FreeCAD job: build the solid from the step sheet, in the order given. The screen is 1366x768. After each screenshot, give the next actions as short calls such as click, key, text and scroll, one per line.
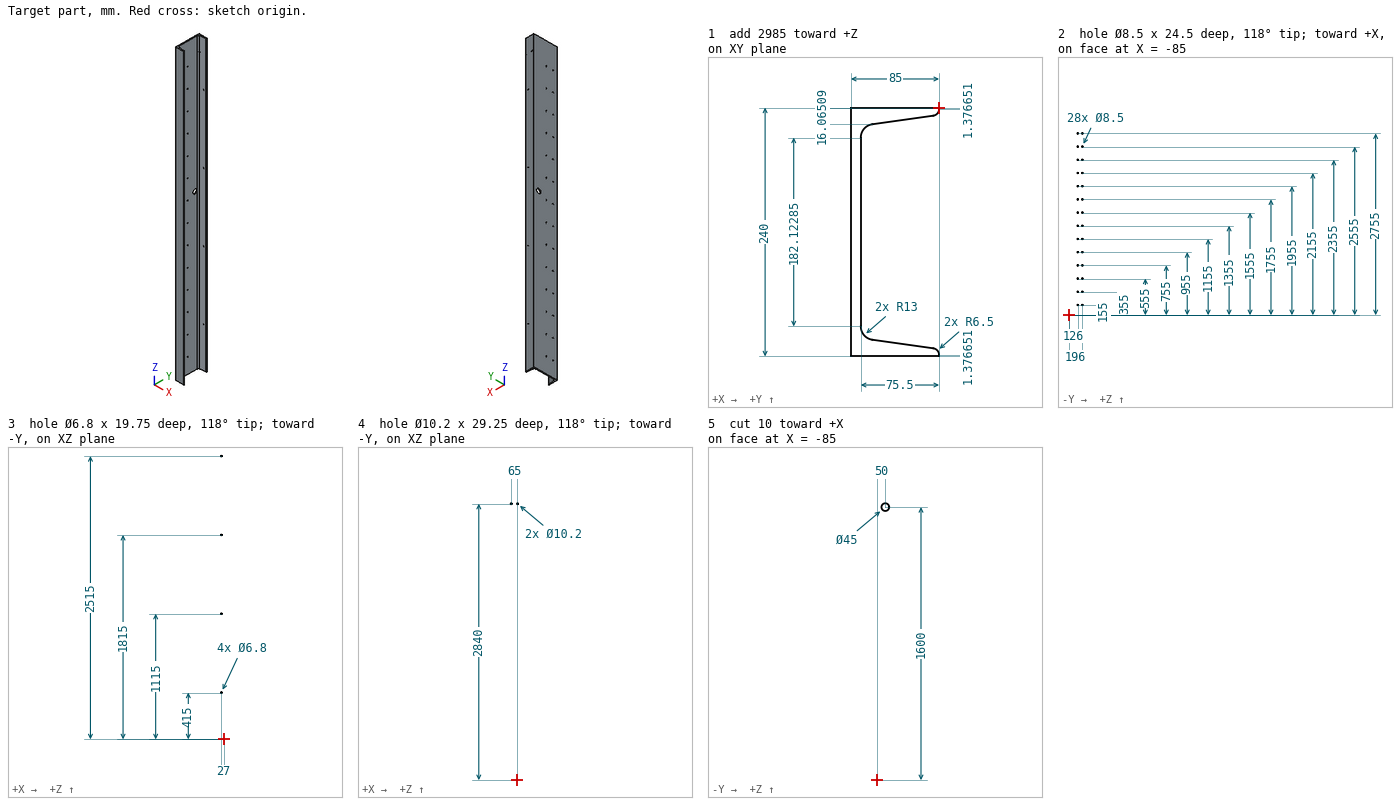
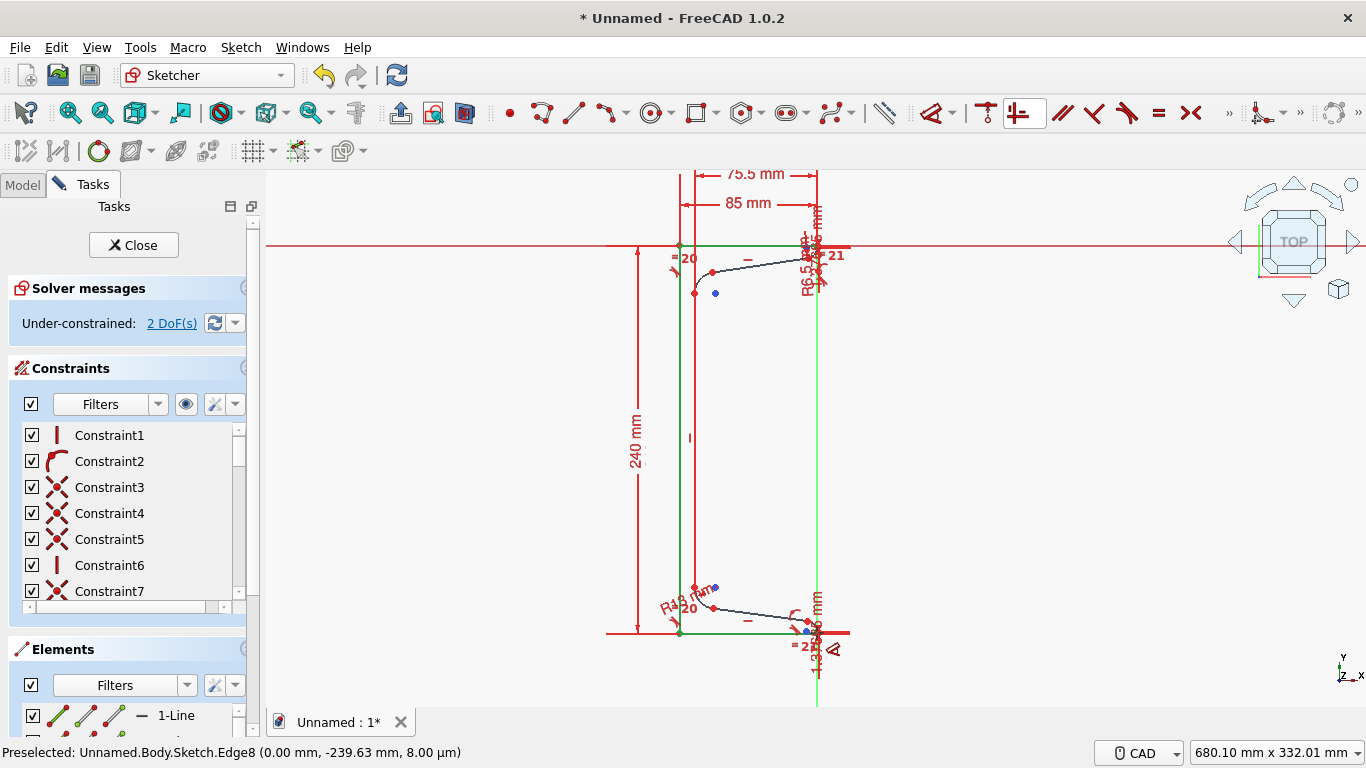
click(695, 499)
click(661, 373)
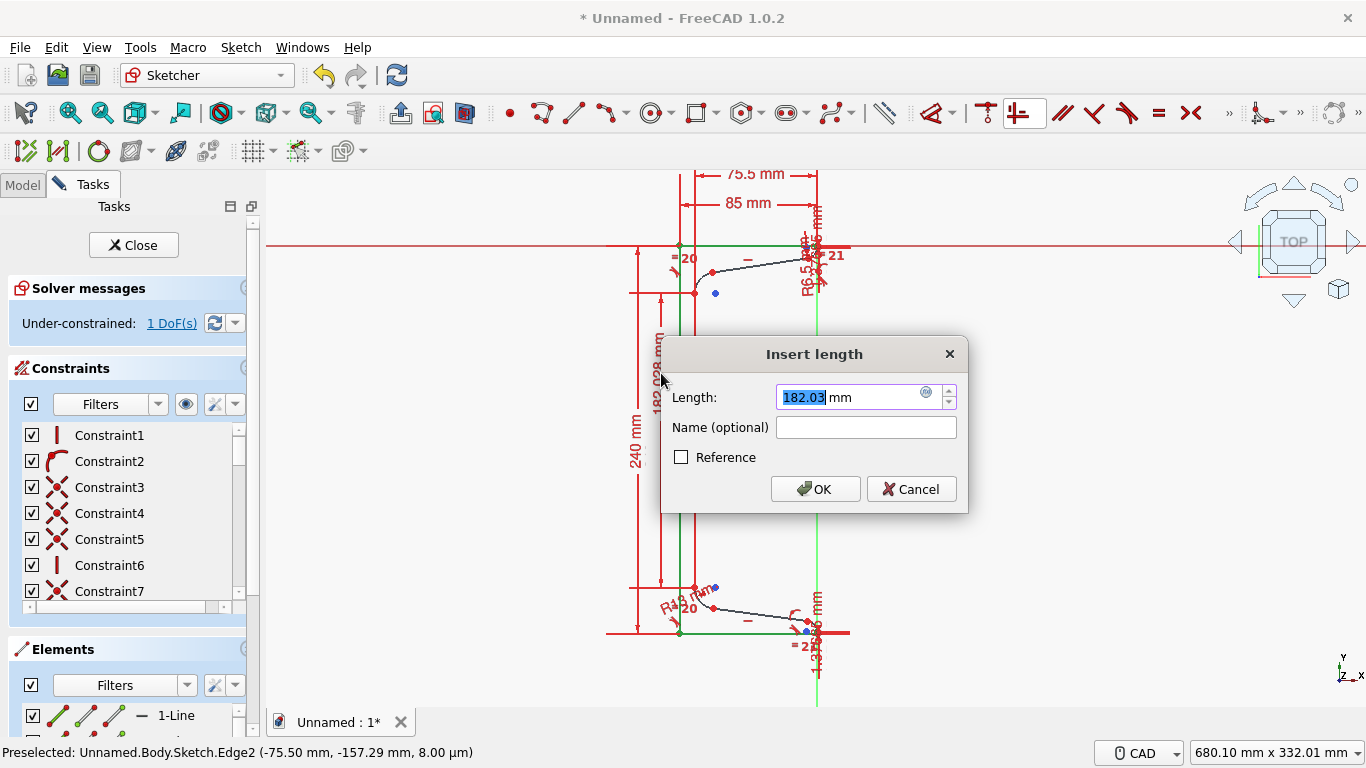
text(182.12285)
key(Return)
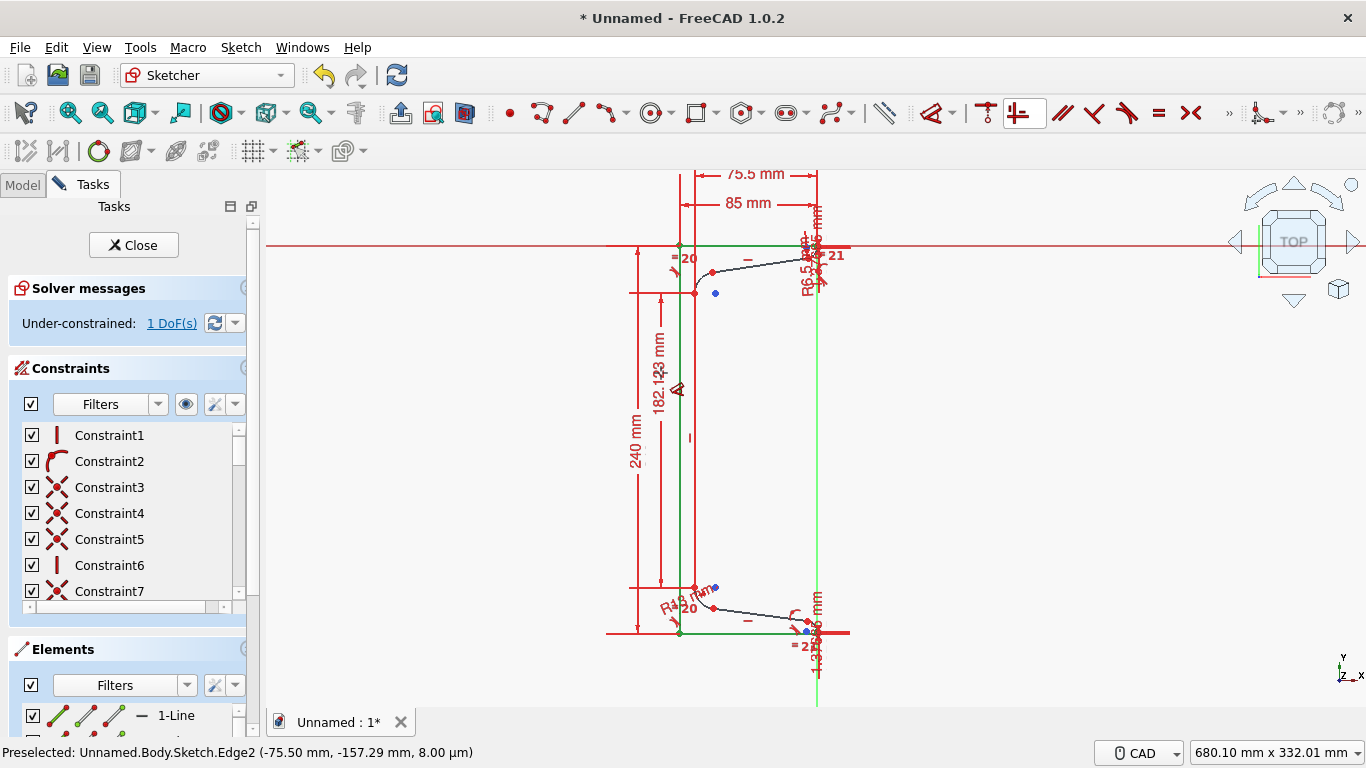
scroll(713, 273, up, 3)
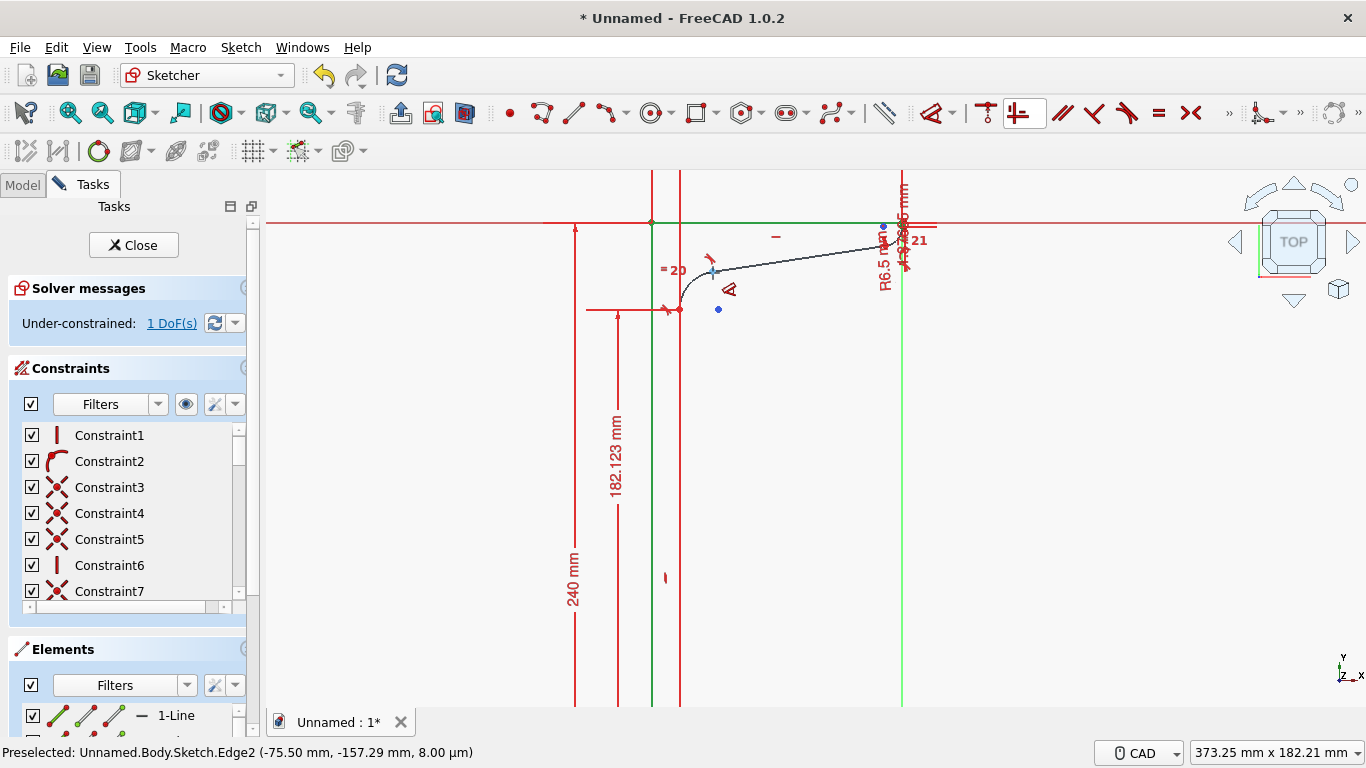
click(712, 272)
click(678, 247)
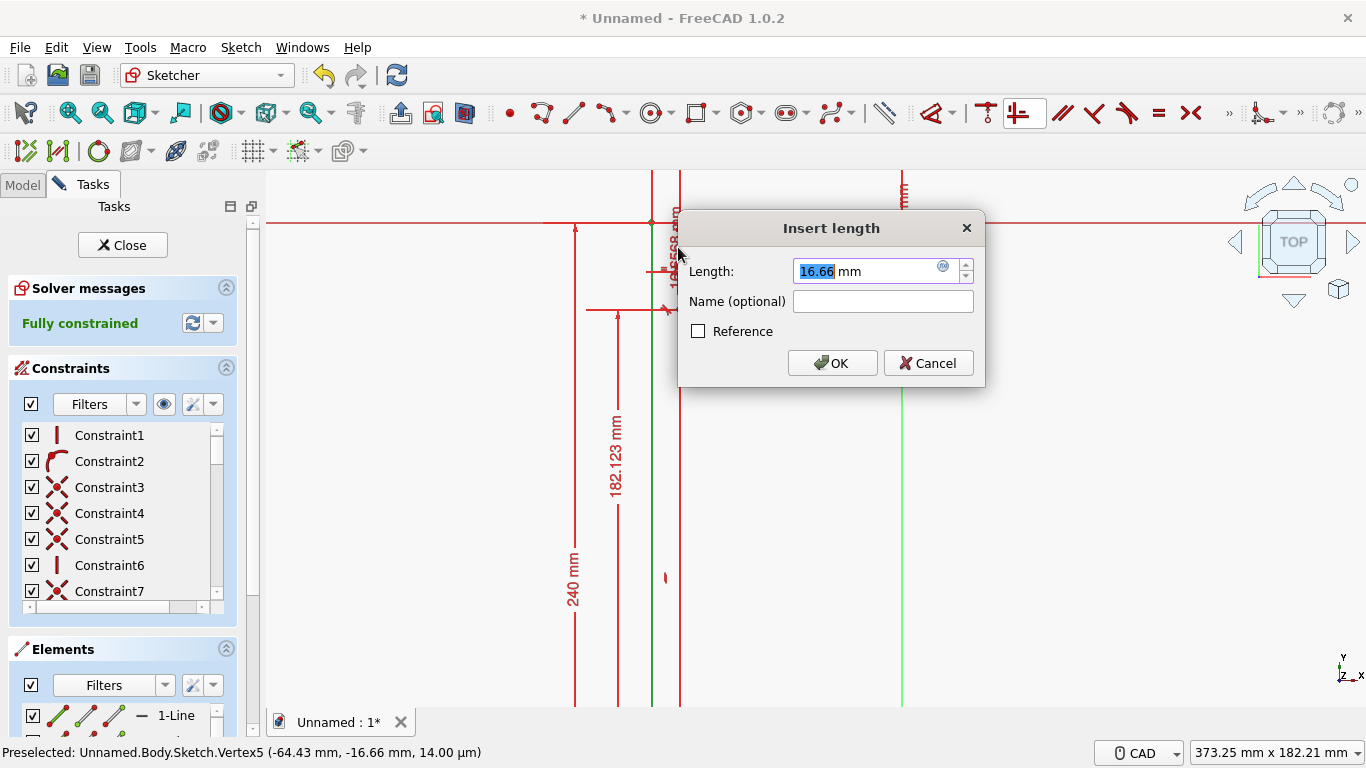
text(16.06509)
key(Return)
key(Escape)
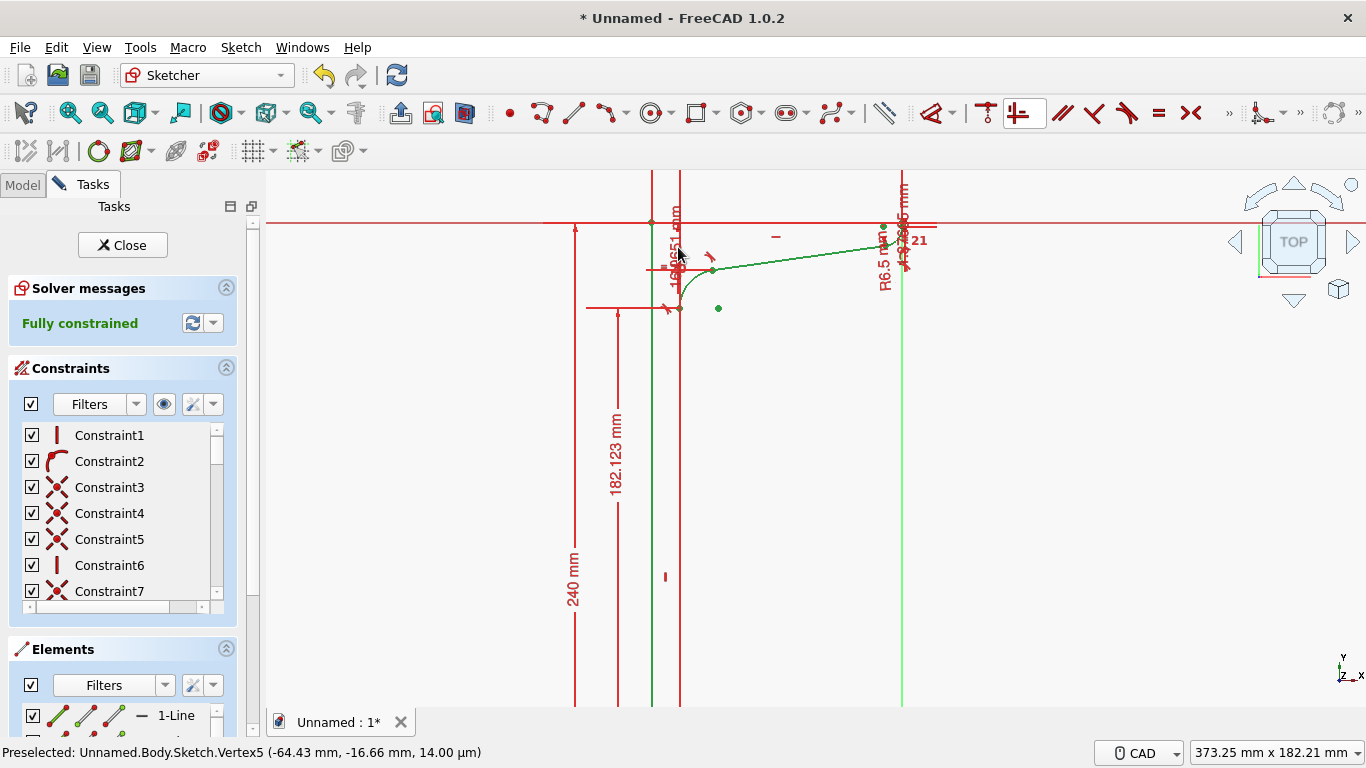
click(123, 245)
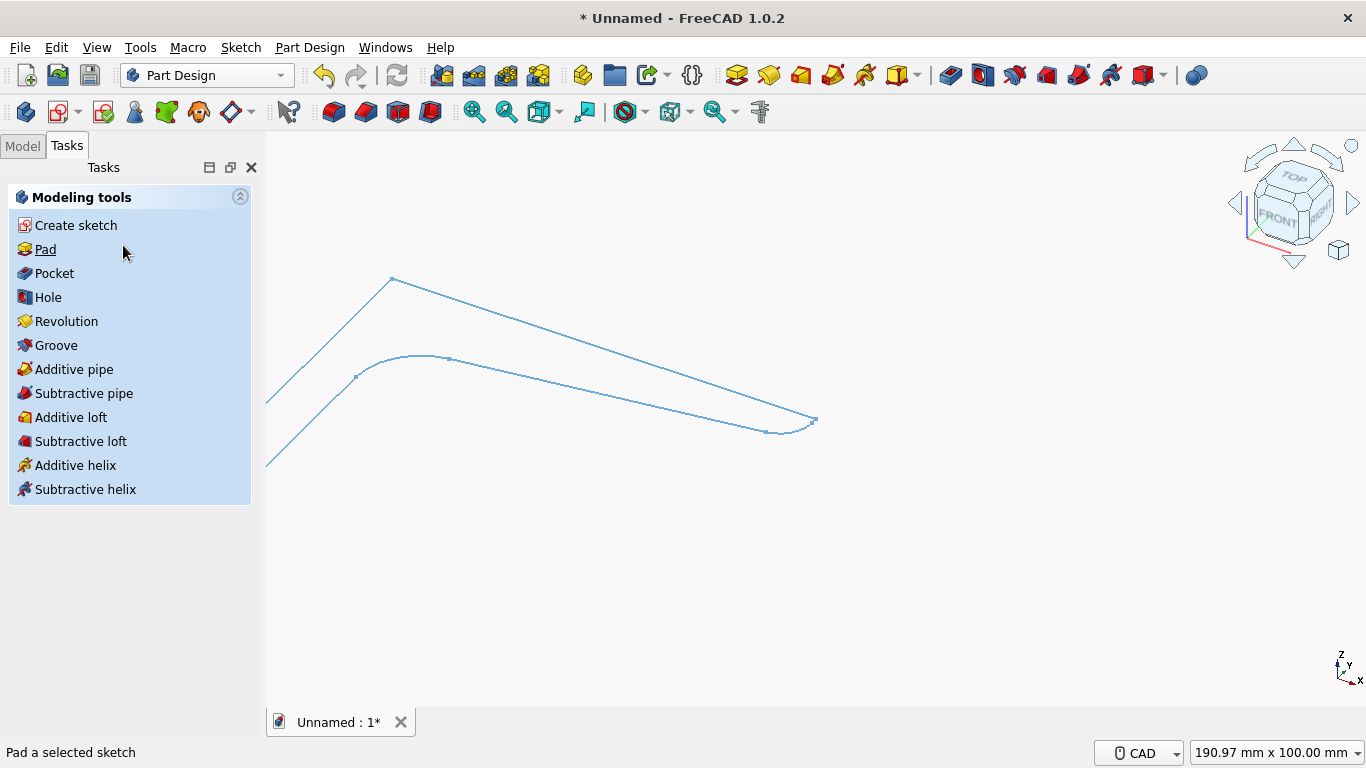
click(738, 76)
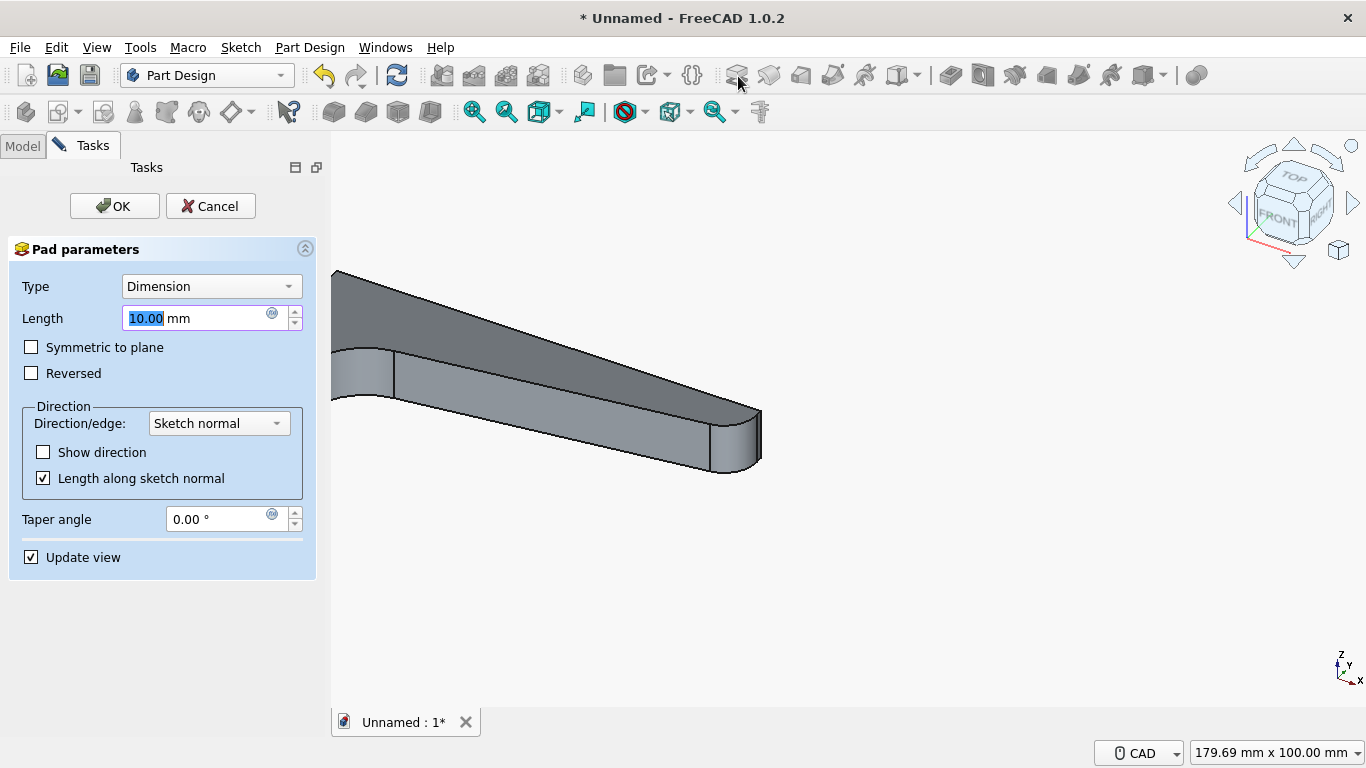
text(2985)
key(Tab)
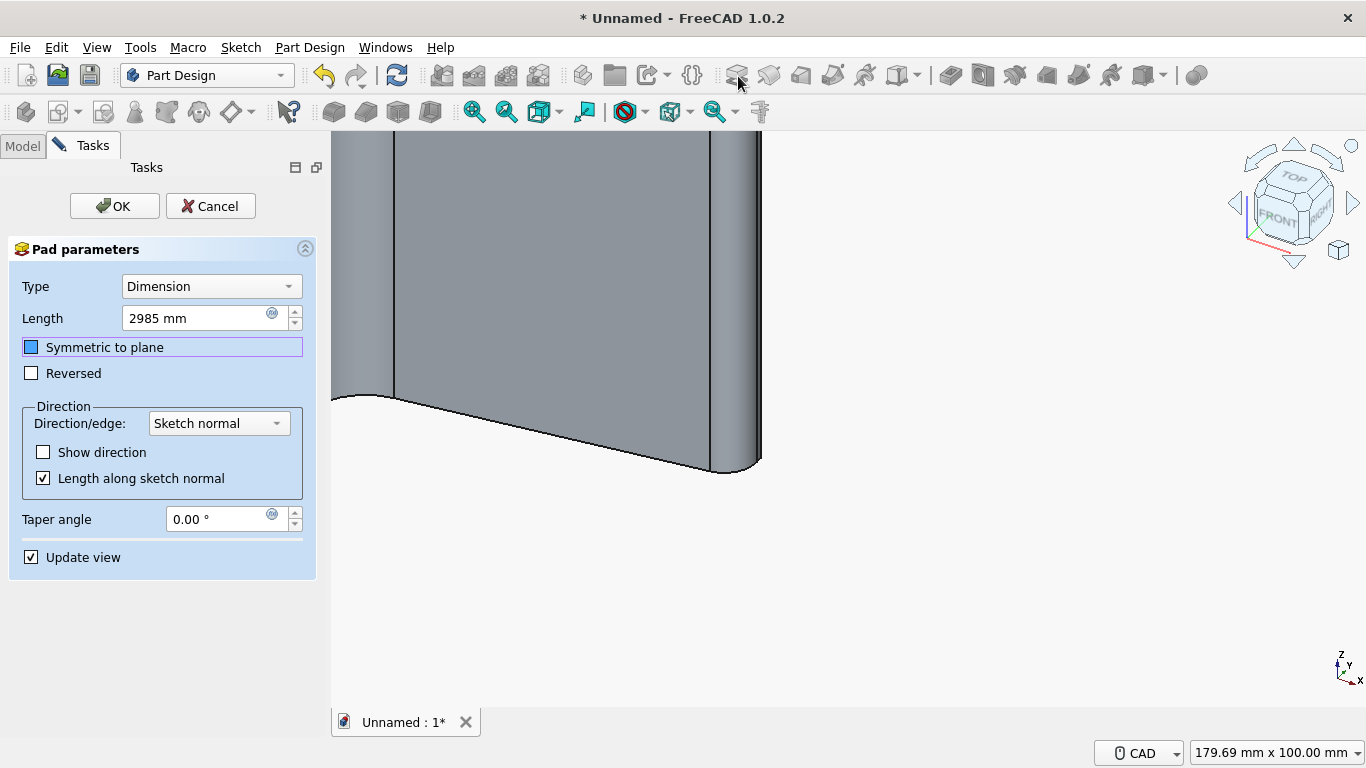
click(115, 206)